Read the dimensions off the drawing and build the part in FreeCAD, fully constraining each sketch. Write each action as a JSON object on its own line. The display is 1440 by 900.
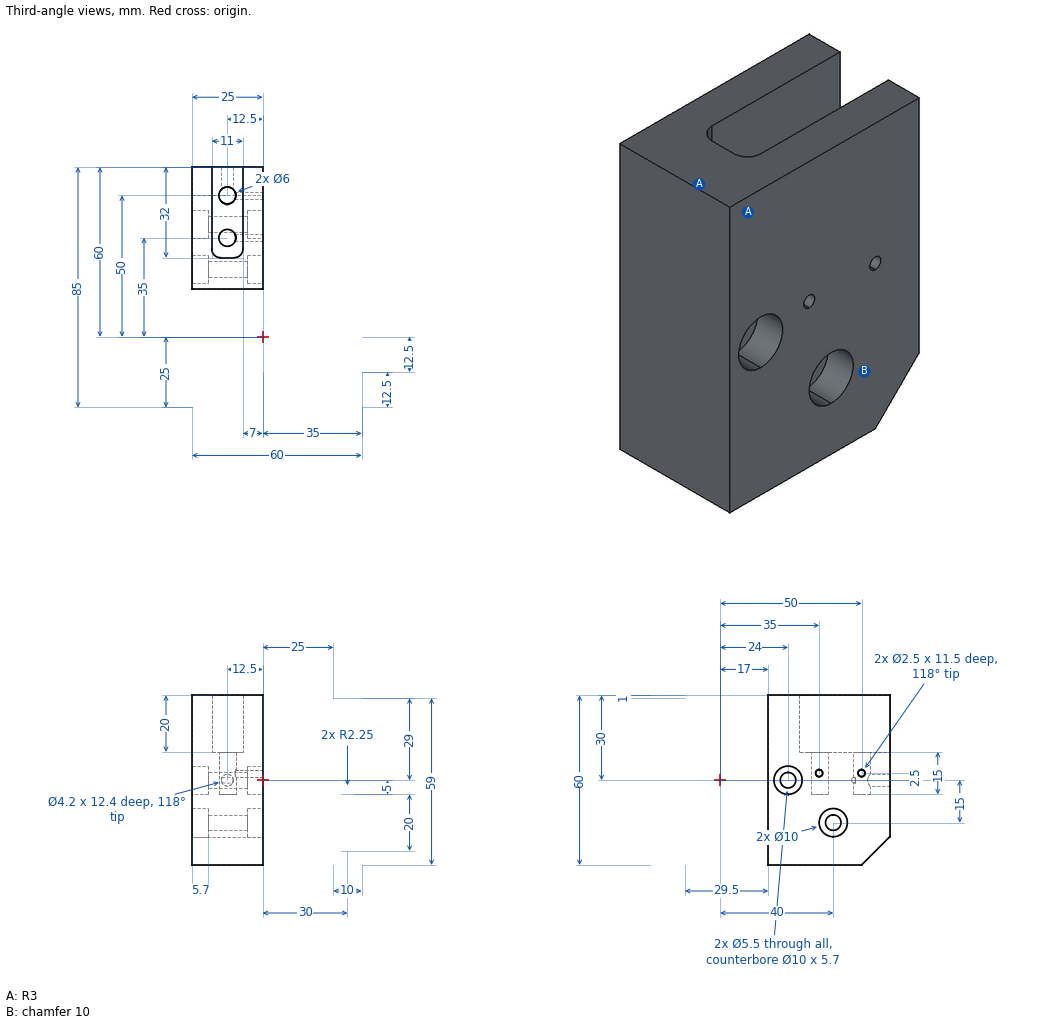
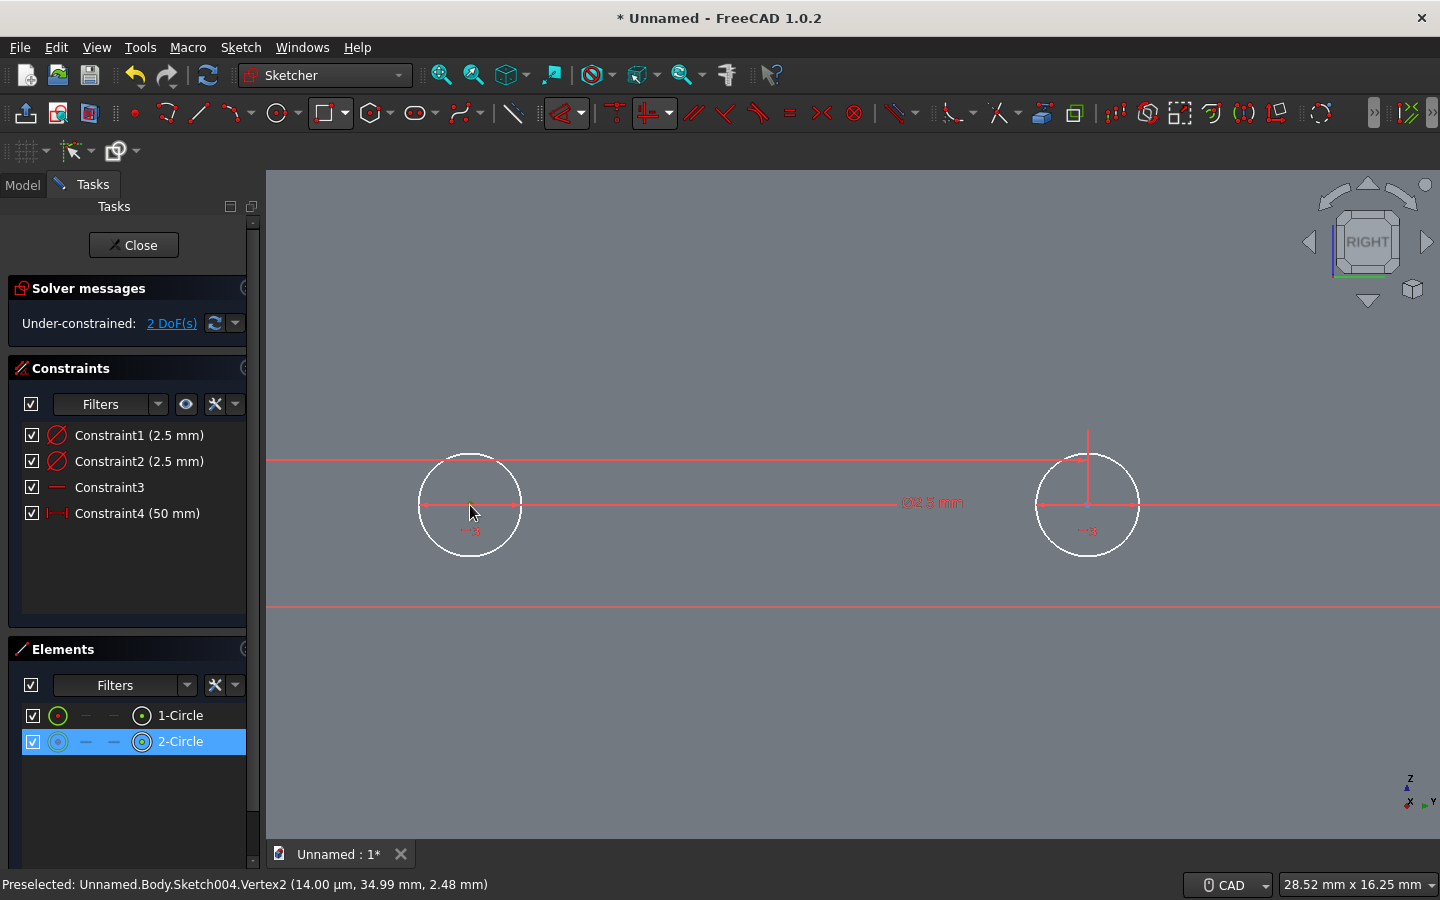
{"action": "left_click", "coordinate": [584, 114]}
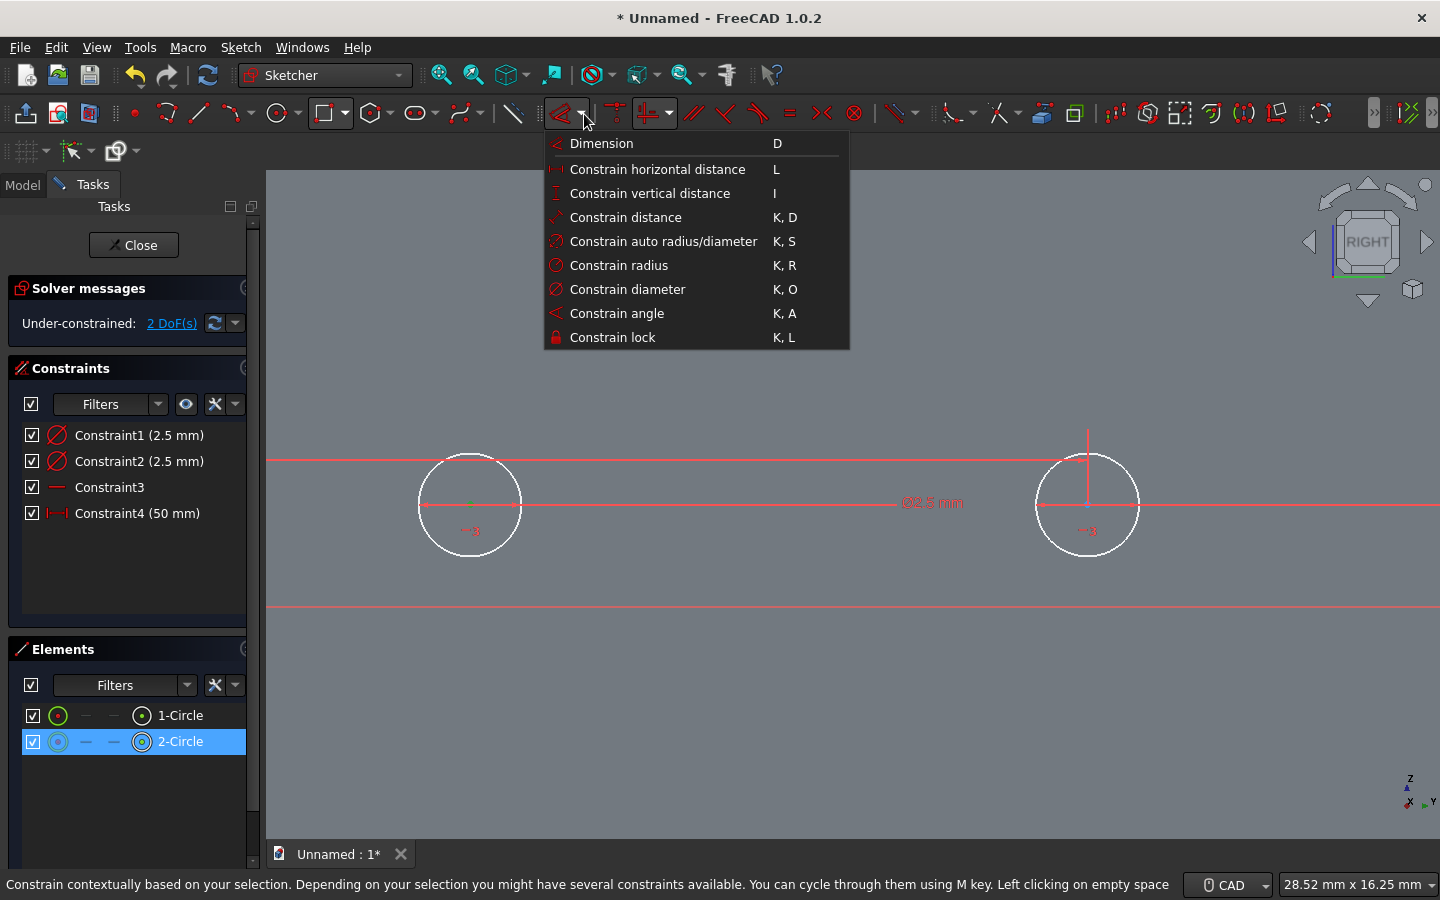
{"action": "left_click", "coordinate": [697, 169]}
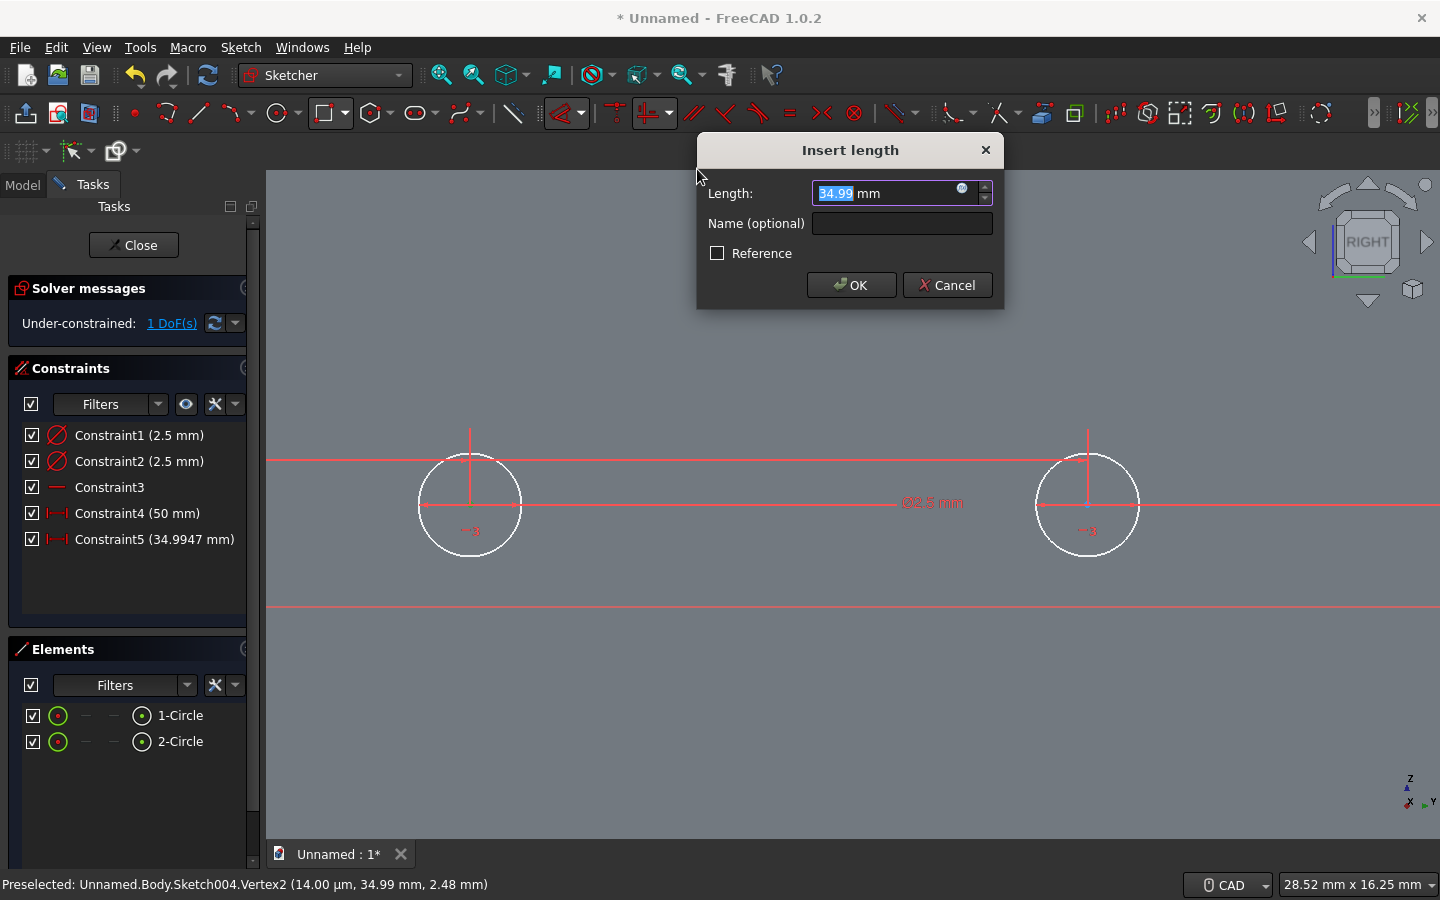
{"action": "type", "text": "35"}
{"action": "key", "text": "Return"}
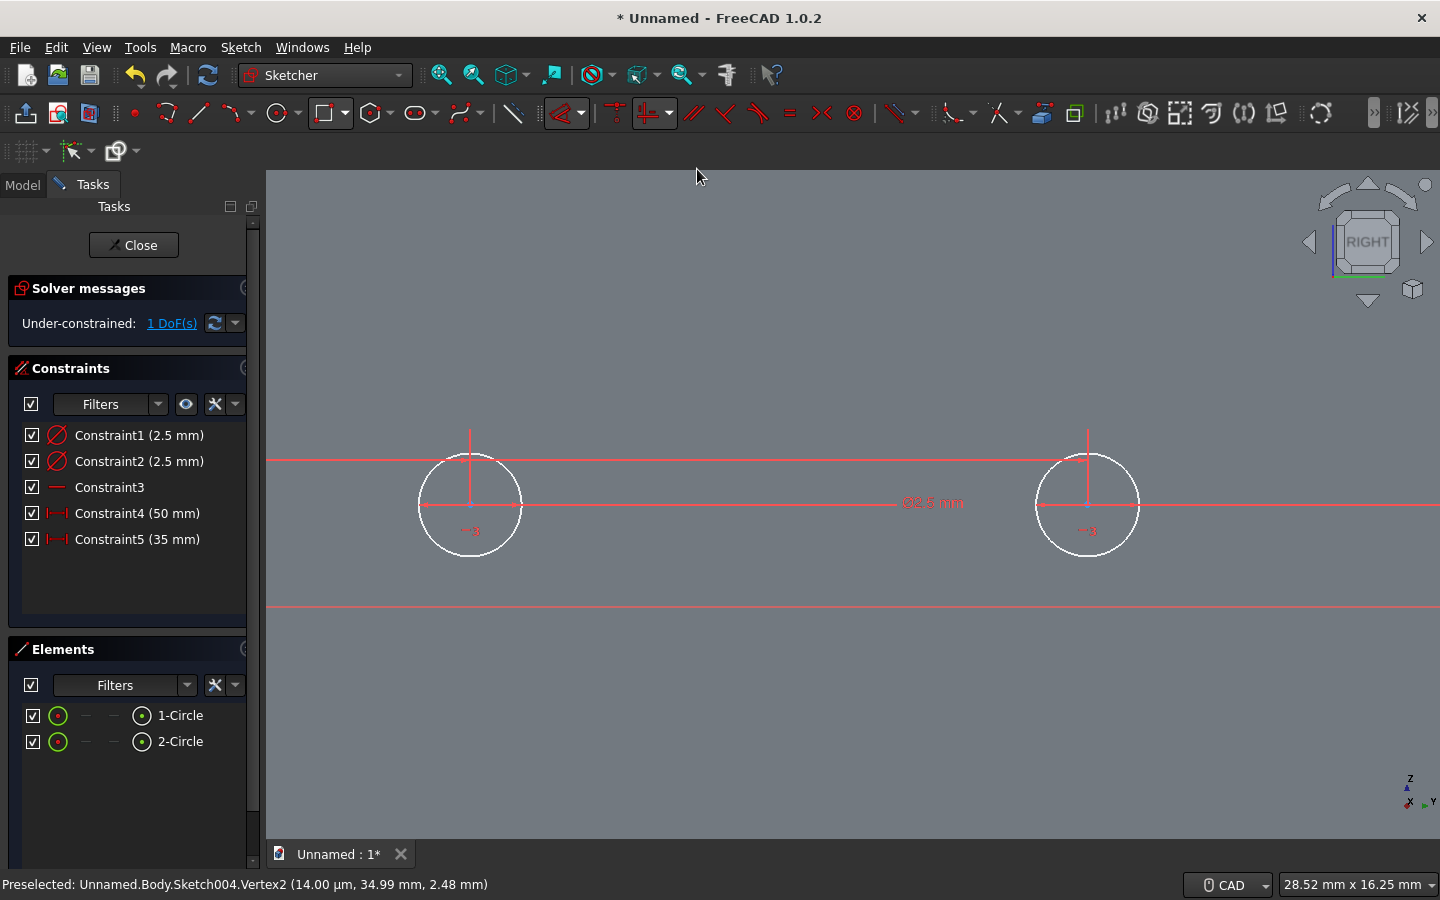
{"action": "left_click", "coordinate": [1088, 505]}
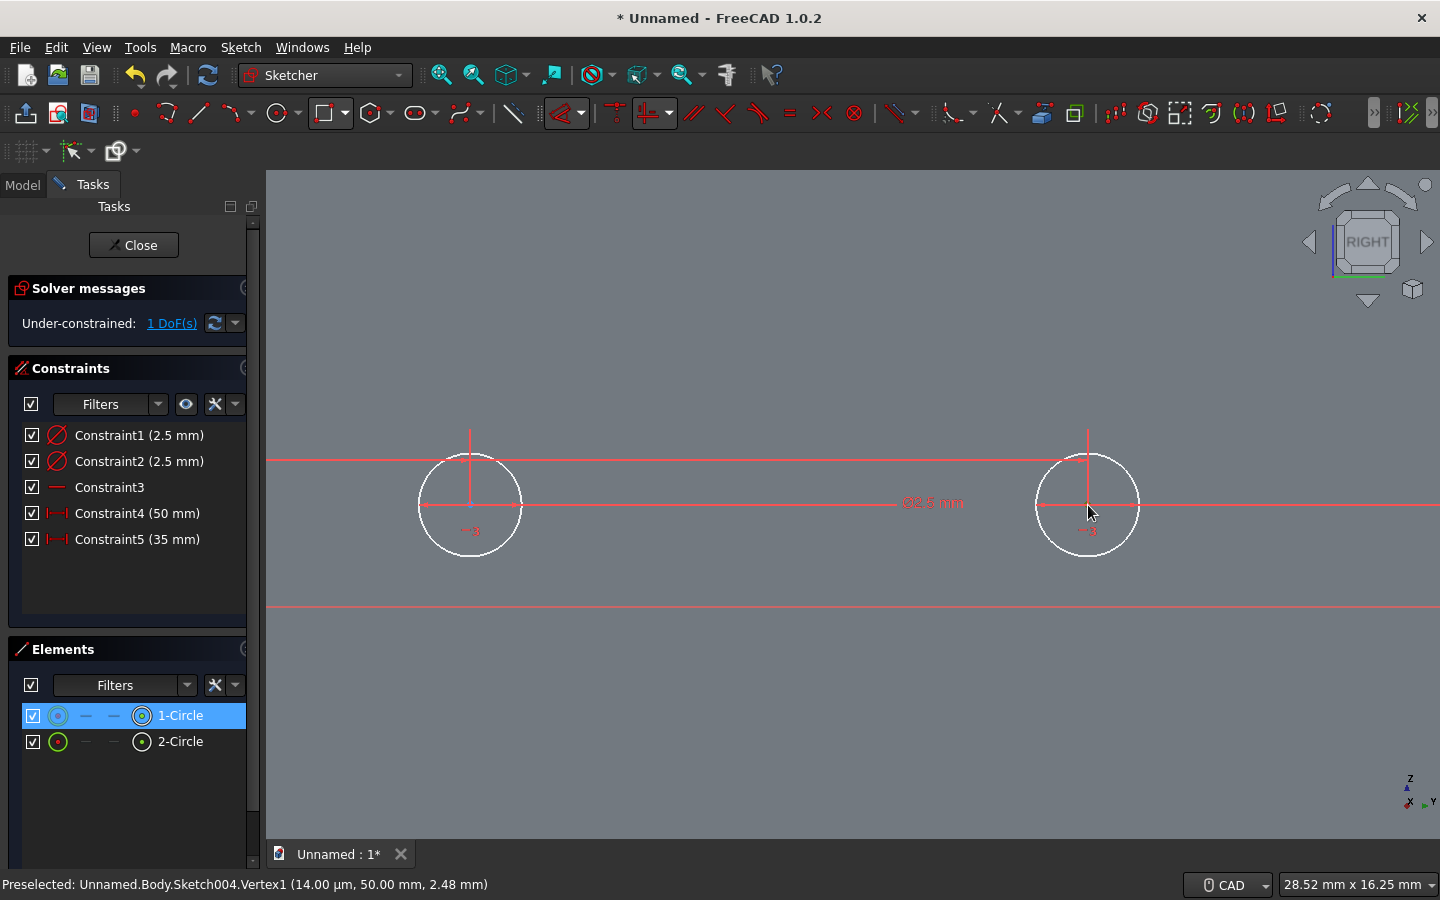
{"action": "left_click", "coordinate": [584, 114]}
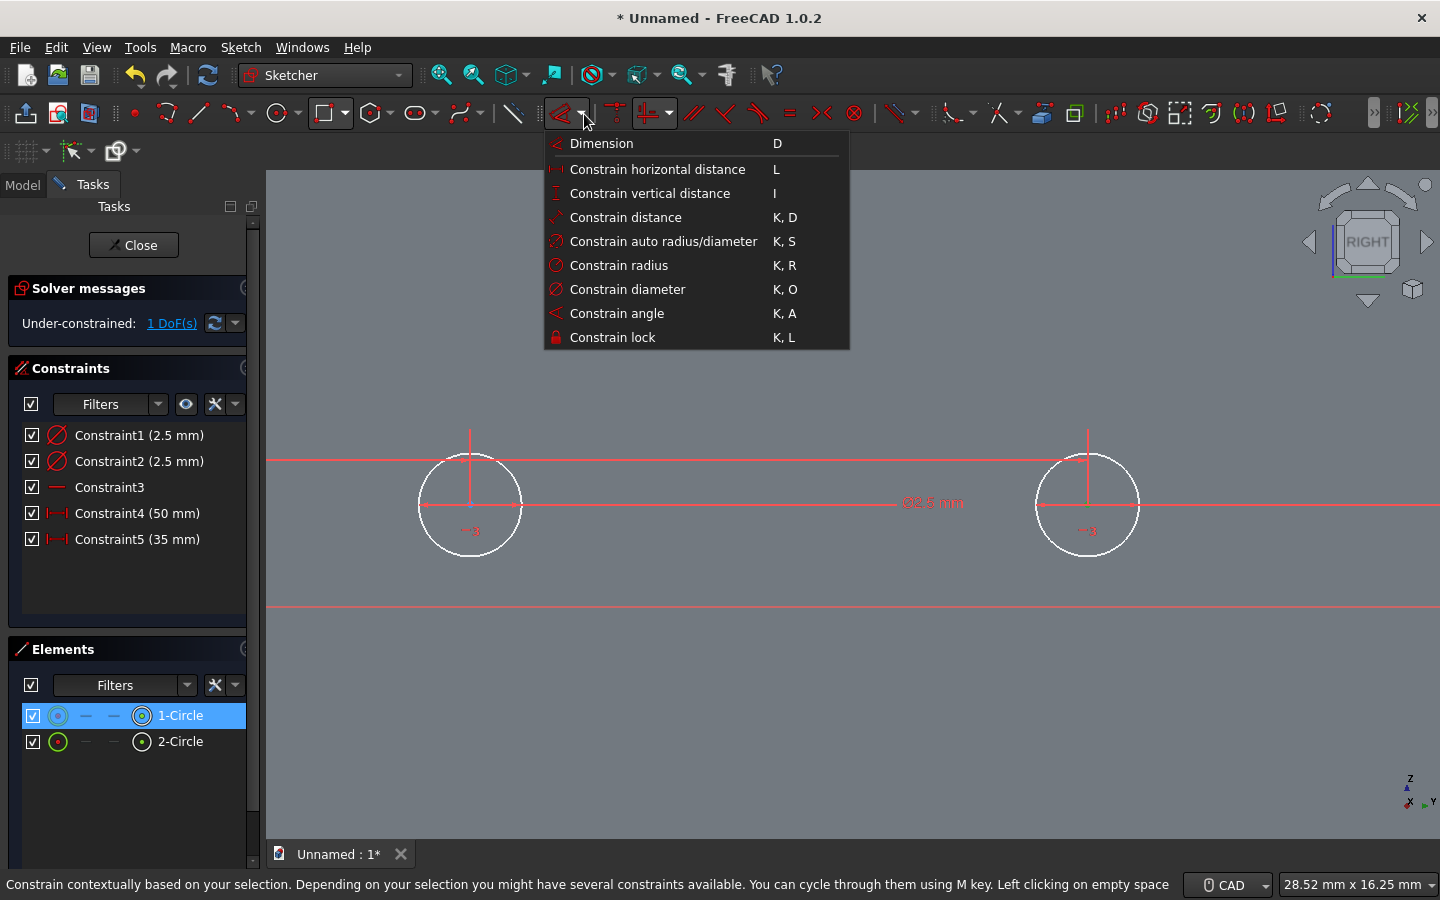
{"action": "left_click", "coordinate": [697, 193]}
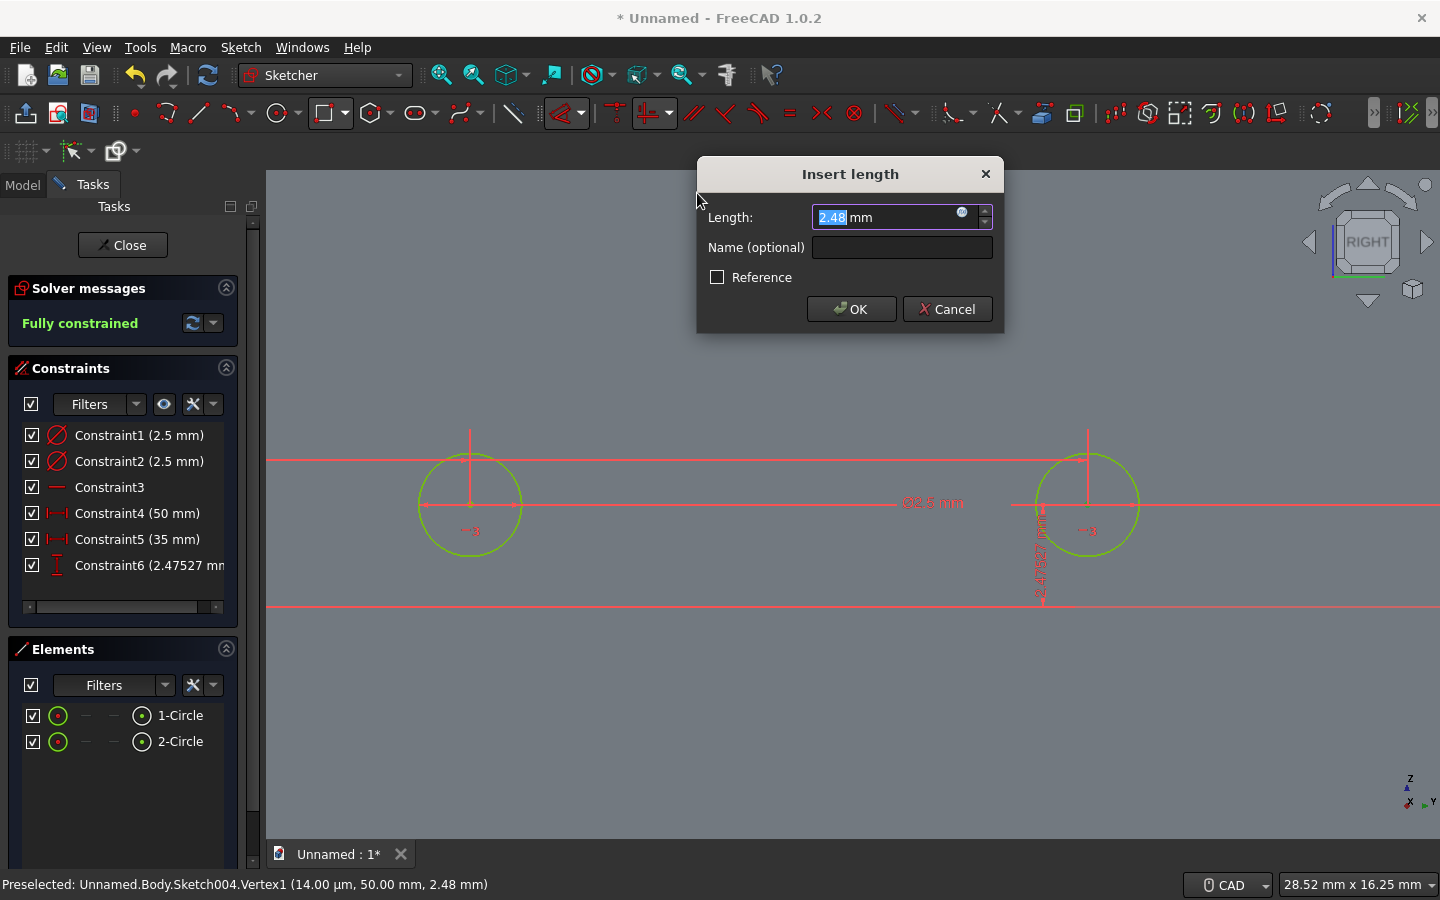
{"action": "type", "text": "2.5"}
{"action": "key", "text": "Return"}